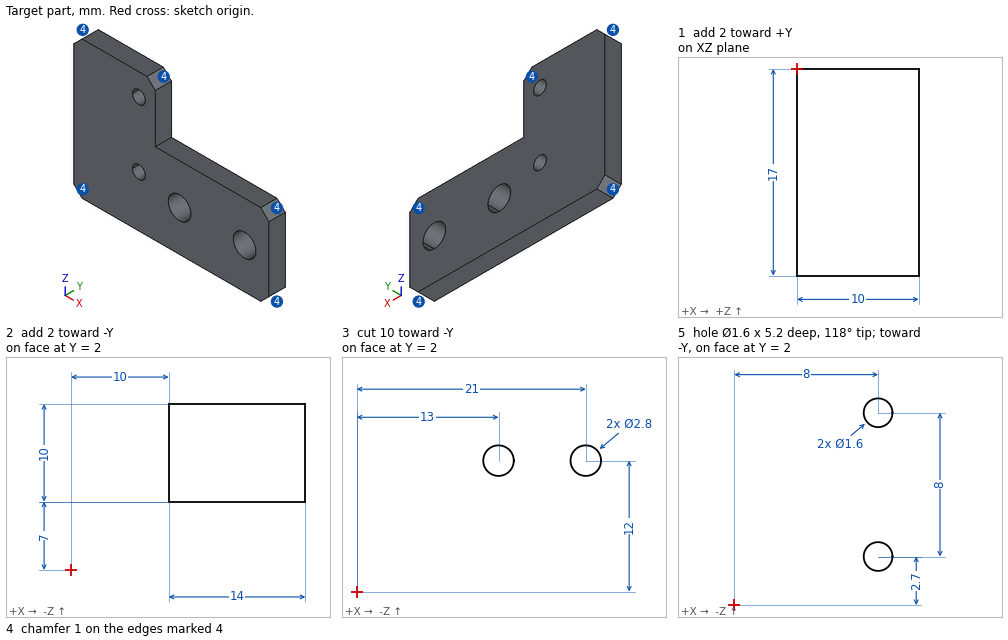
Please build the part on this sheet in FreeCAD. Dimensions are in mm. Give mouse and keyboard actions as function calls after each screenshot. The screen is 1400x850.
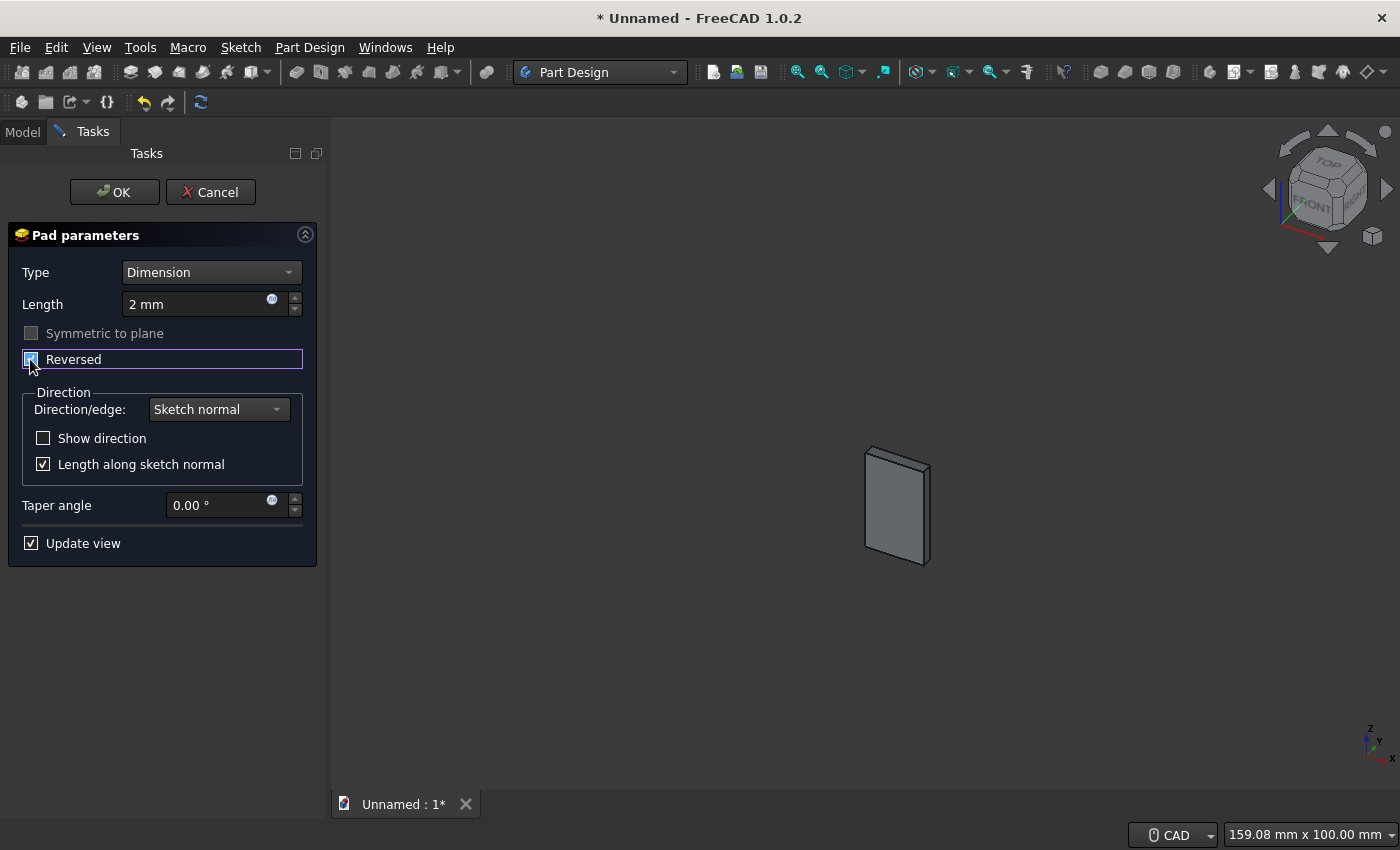
click(115, 192)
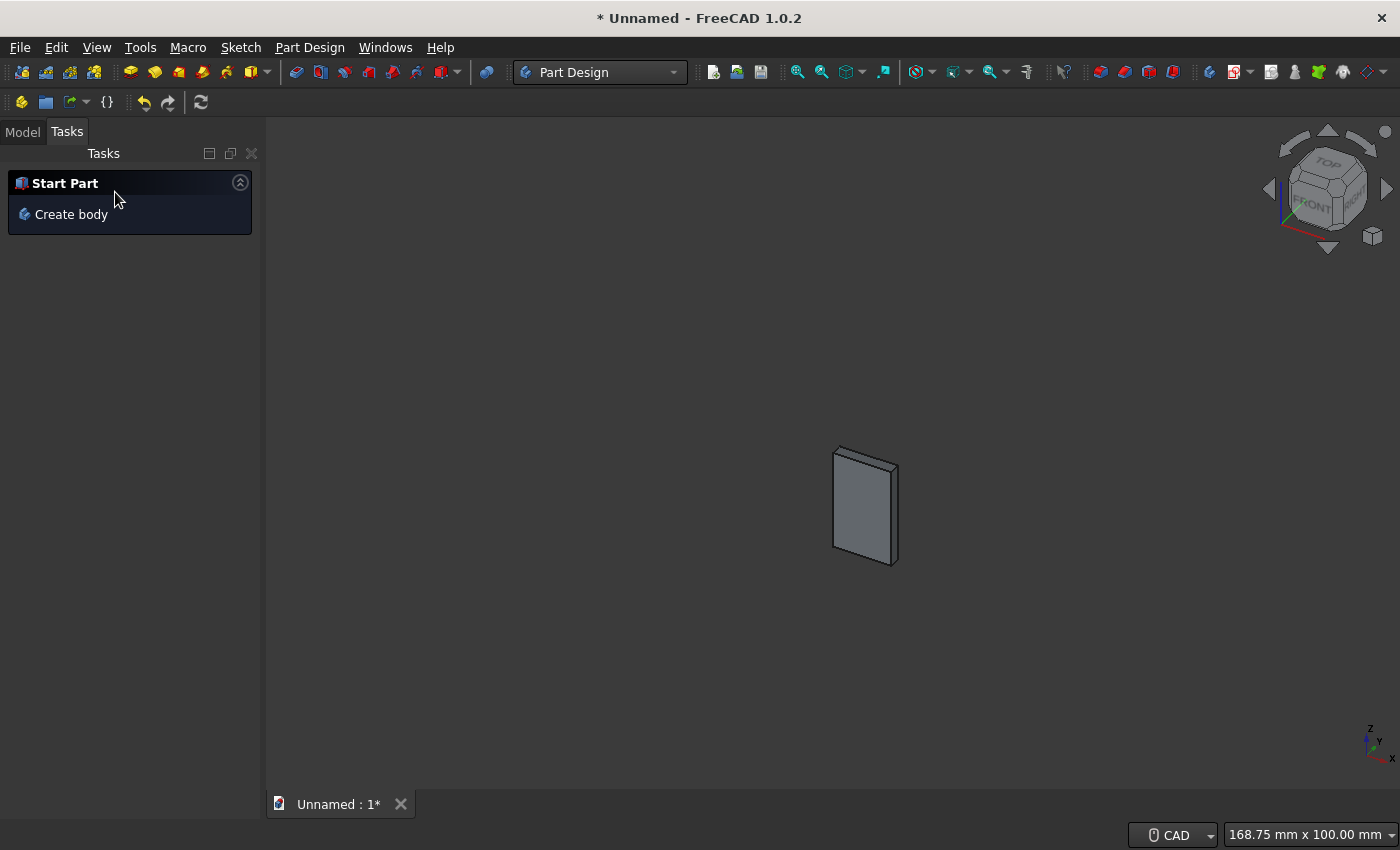
click(798, 72)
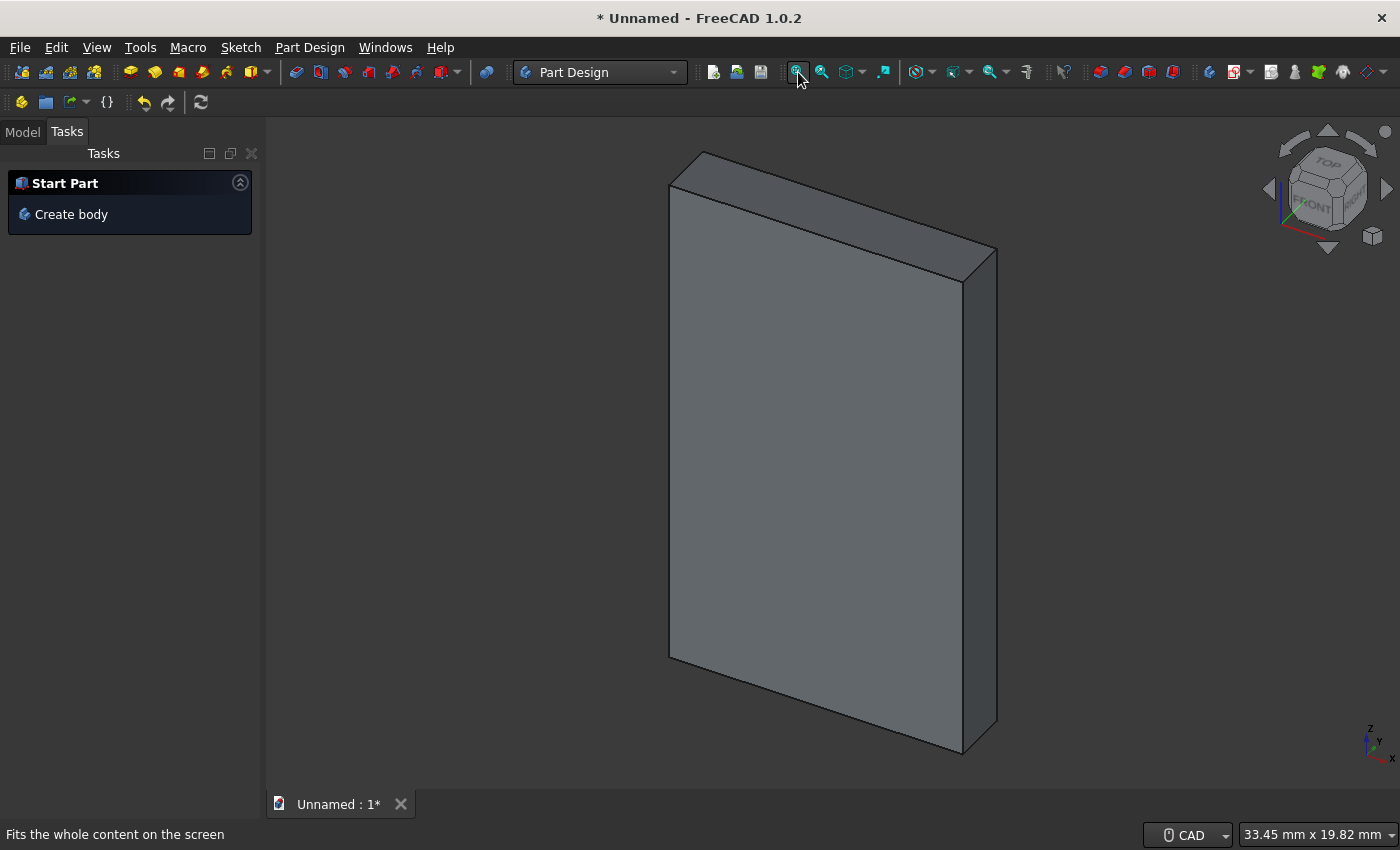
key(4)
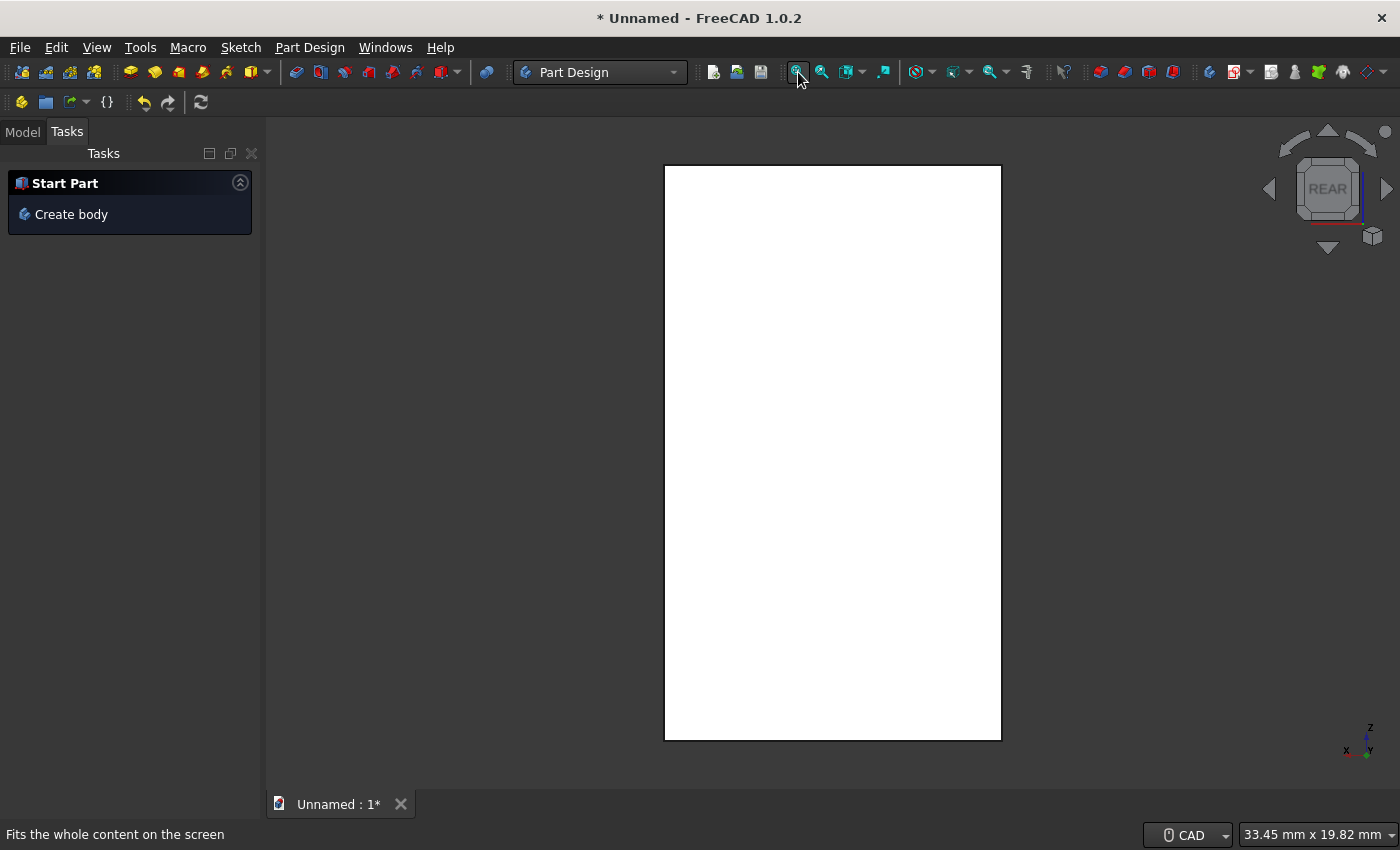
click(833, 370)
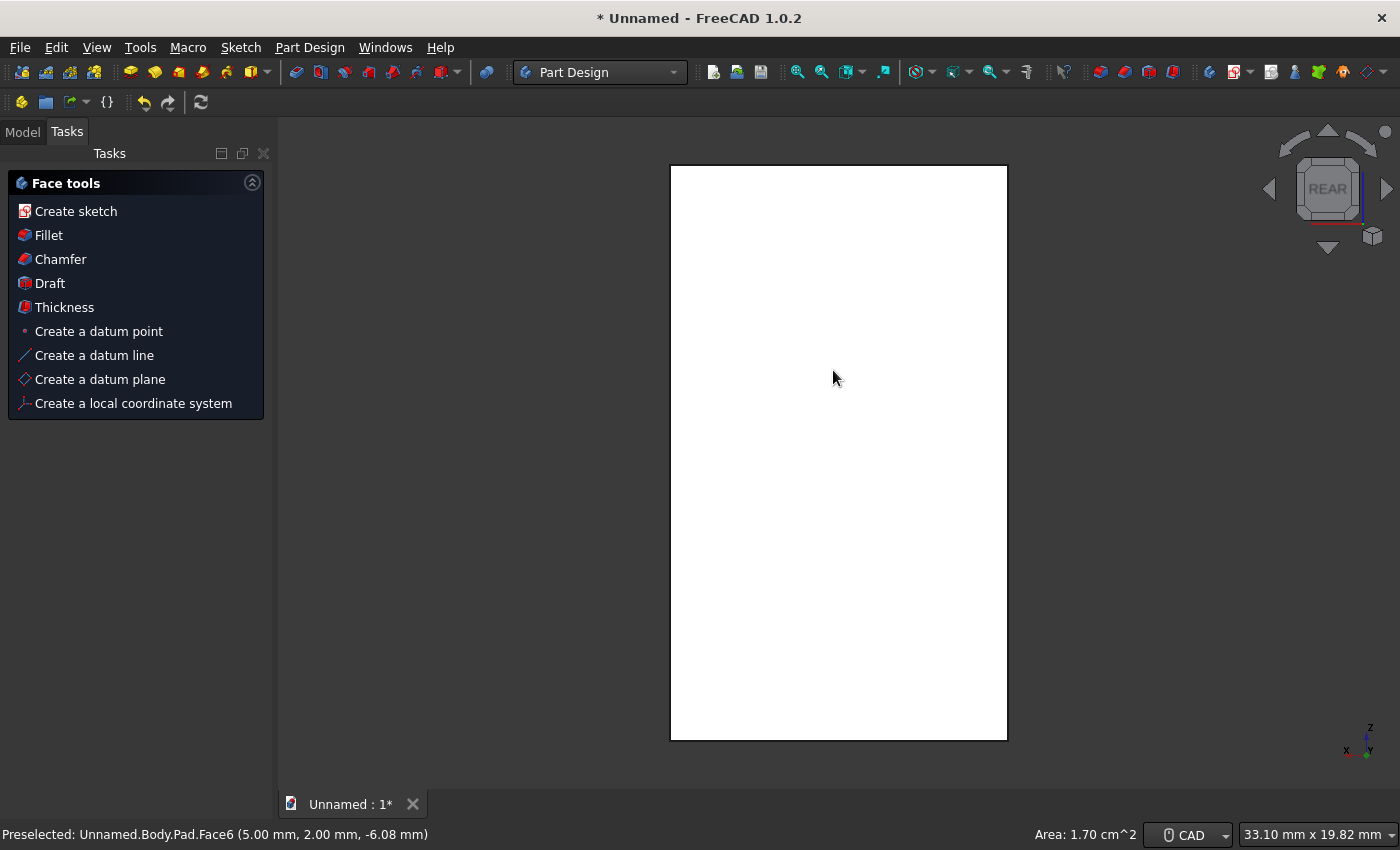
click(1234, 72)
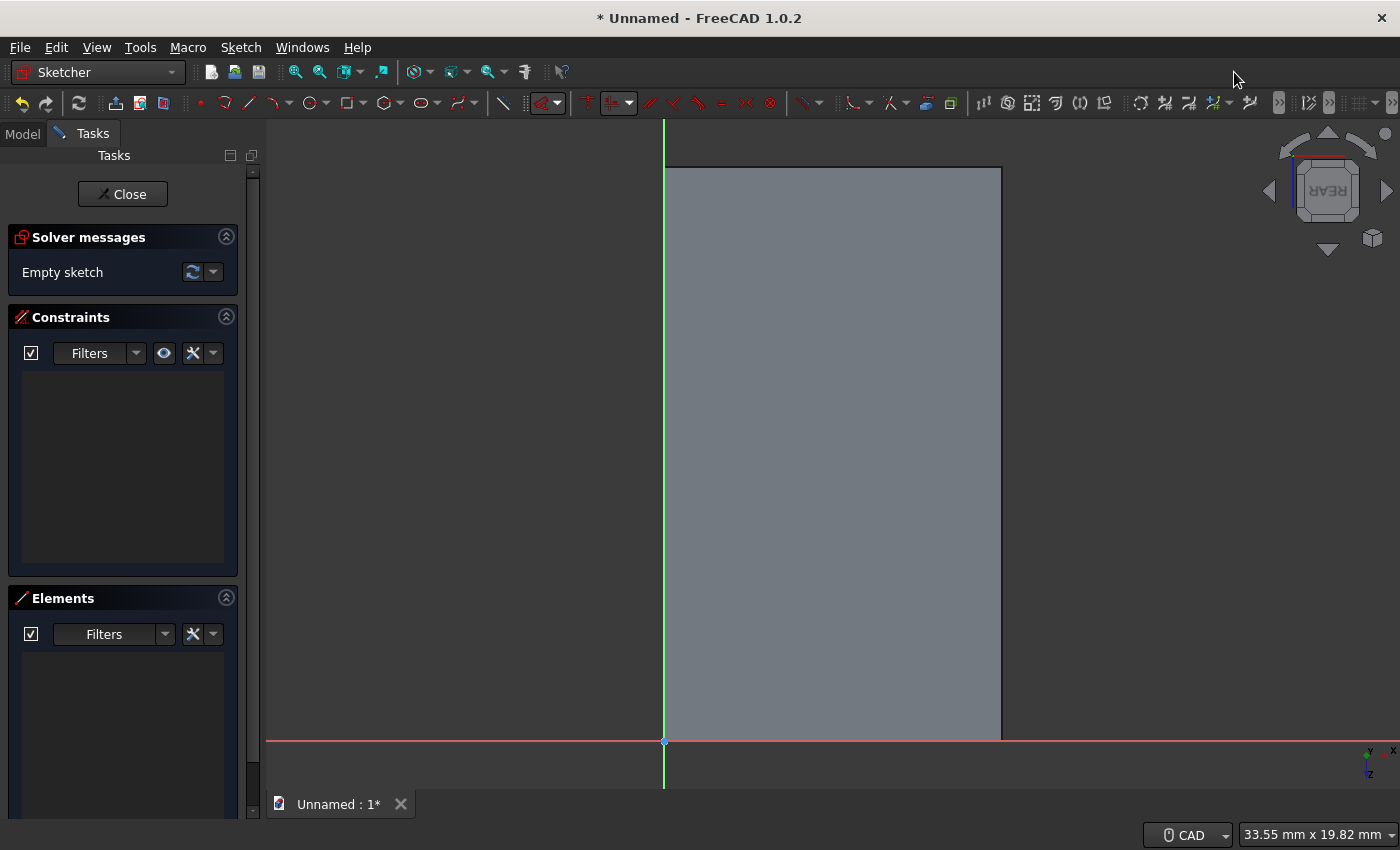
scroll(294, 454, down, 2)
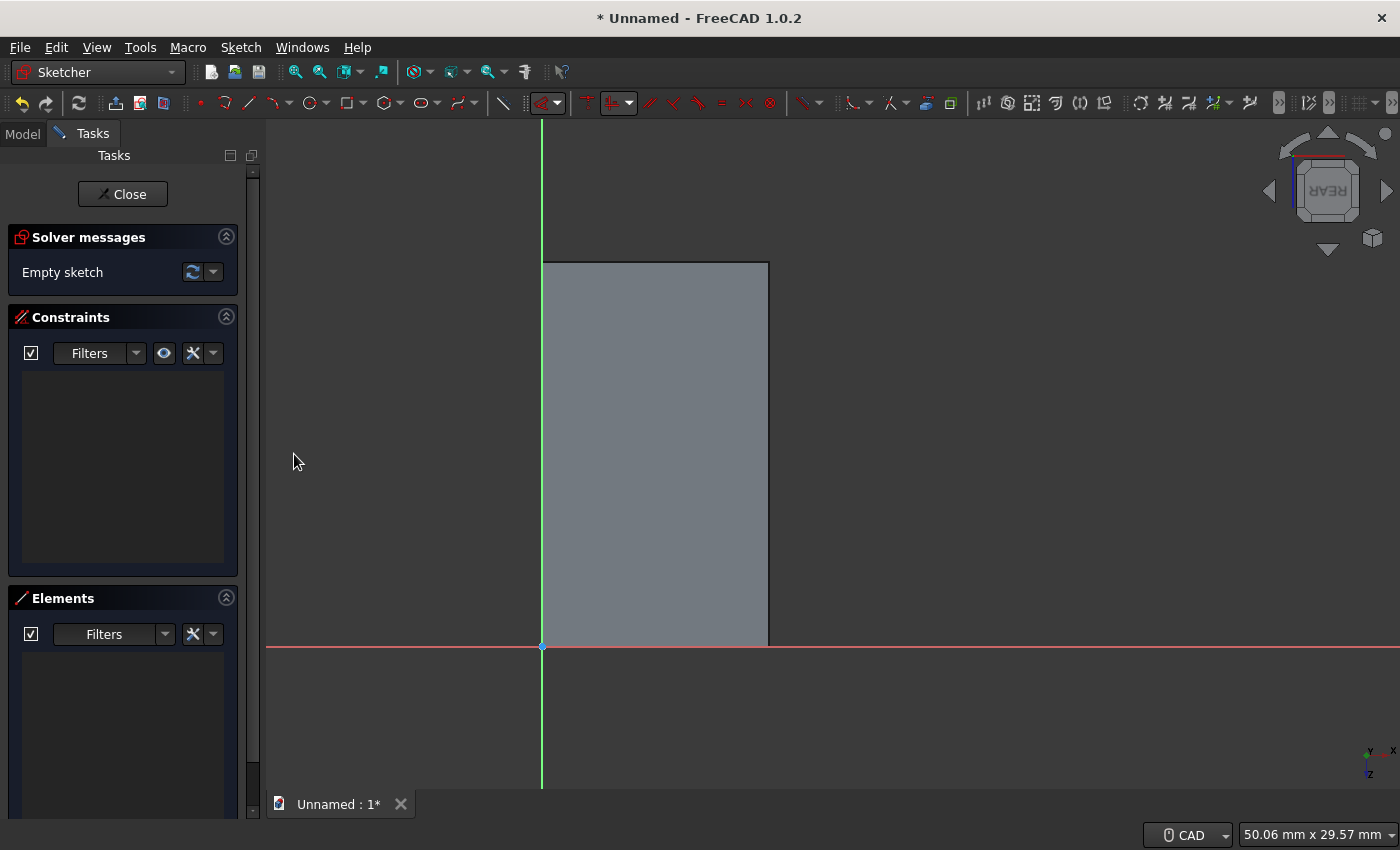
click(348, 104)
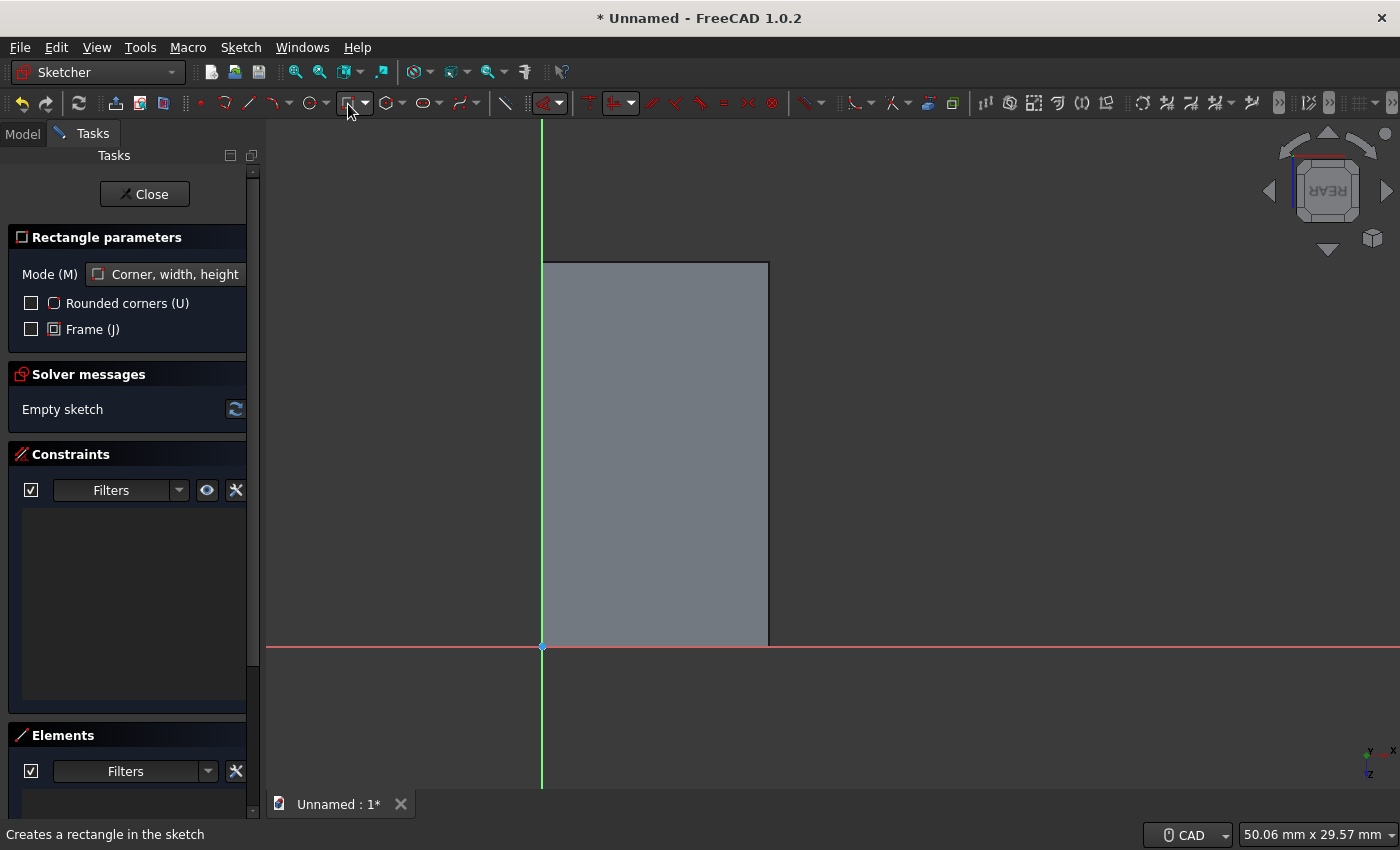
click(769, 262)
click(1086, 488)
key(Escape)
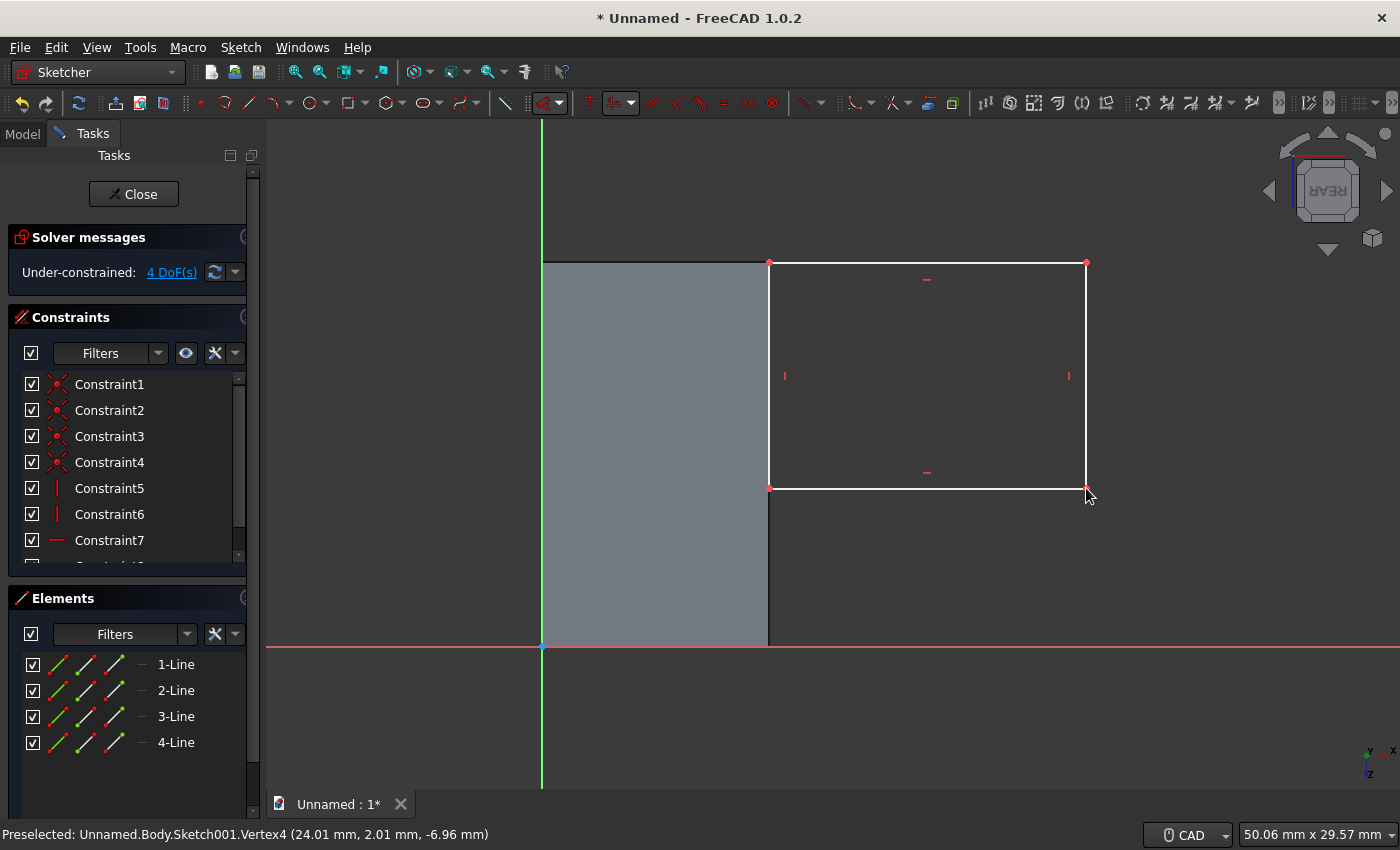
click(769, 331)